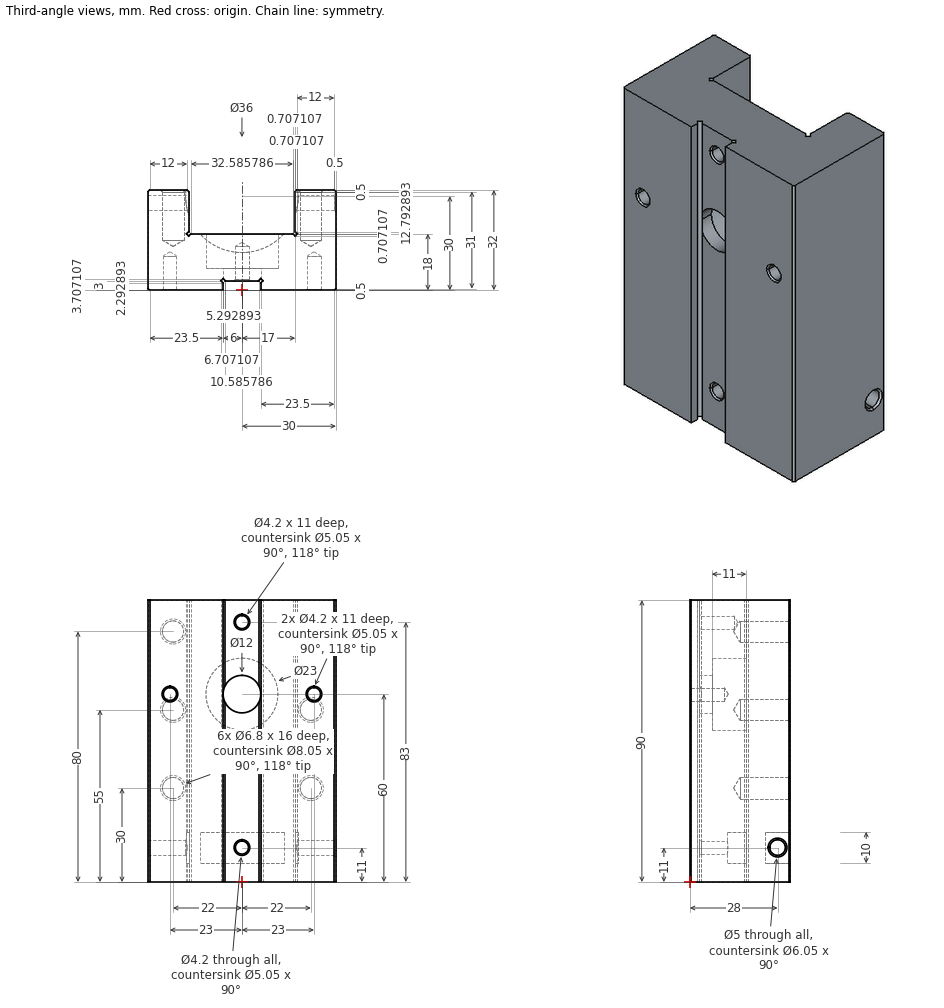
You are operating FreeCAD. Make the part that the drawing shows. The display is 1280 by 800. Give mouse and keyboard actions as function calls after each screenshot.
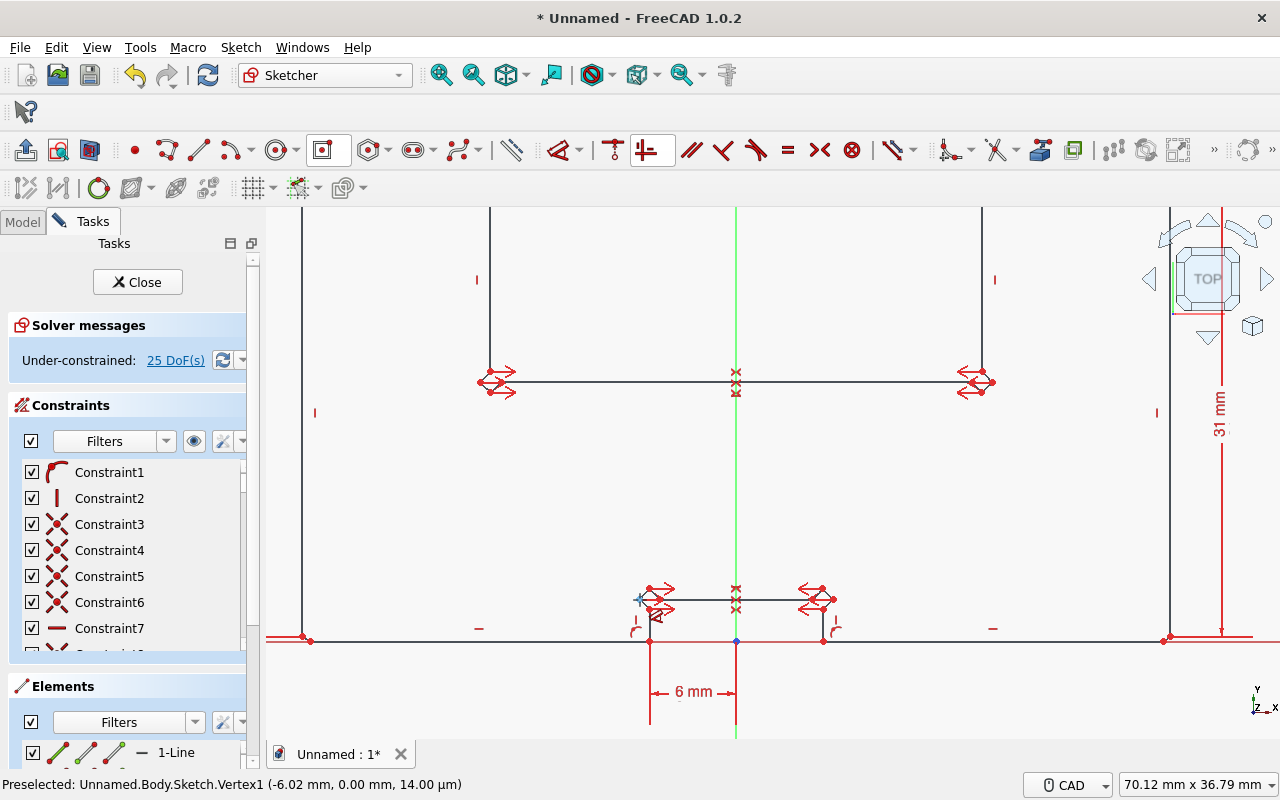
click(640, 600)
click(606, 621)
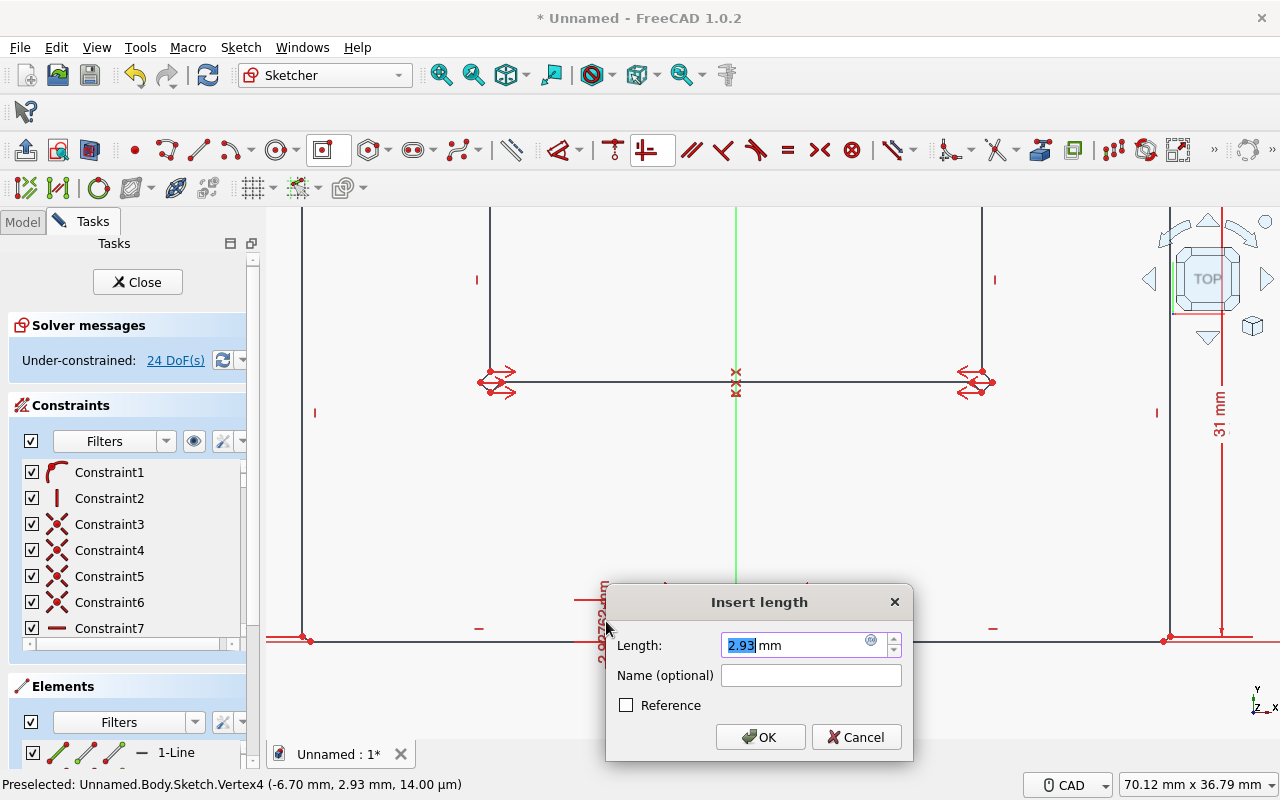
text(3)
key(Return)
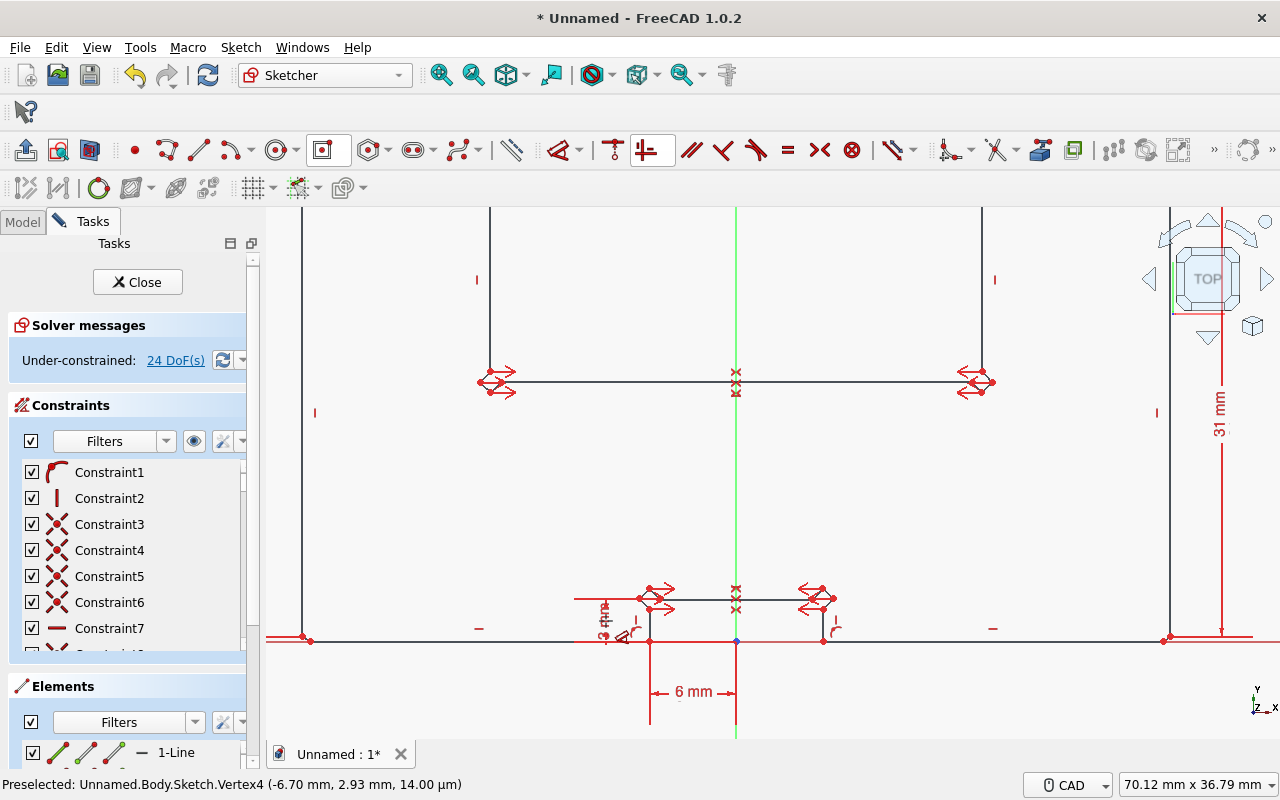
click(650, 589)
click(693, 555)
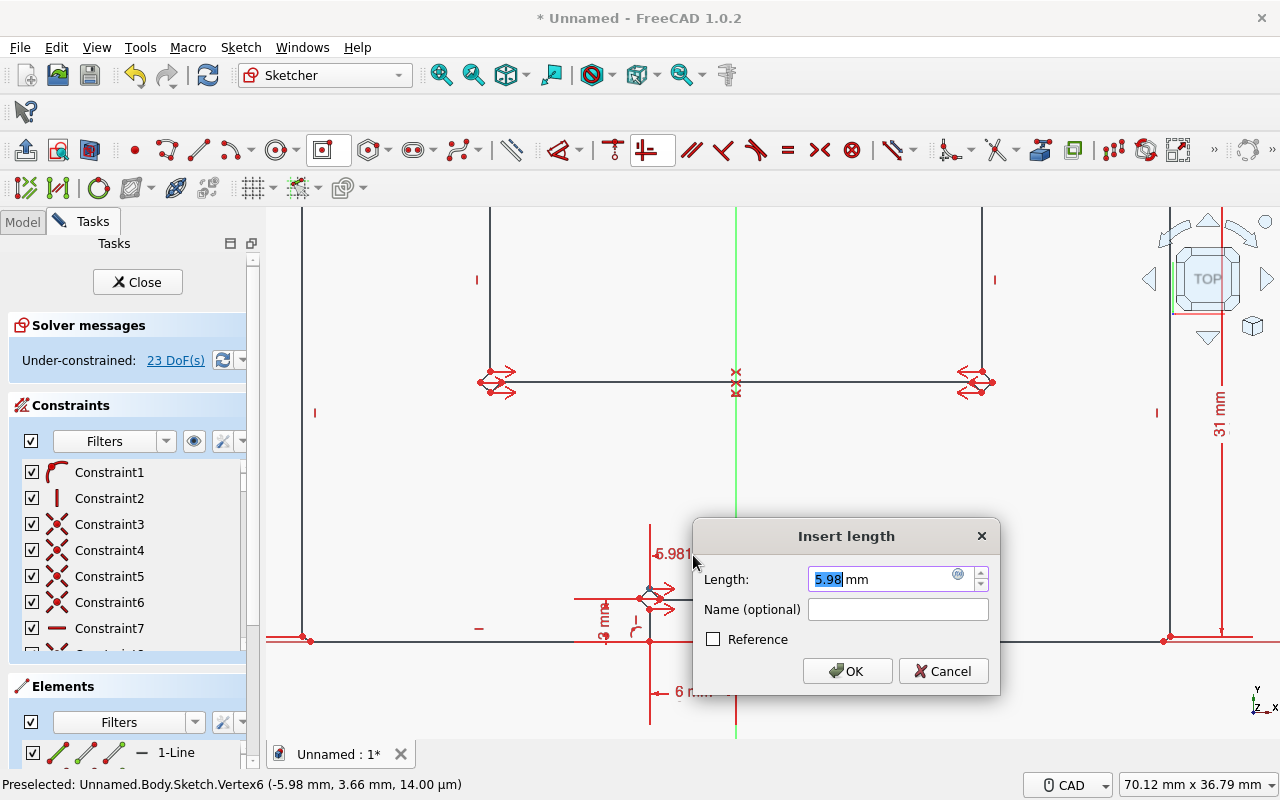
text(6)
key(Return)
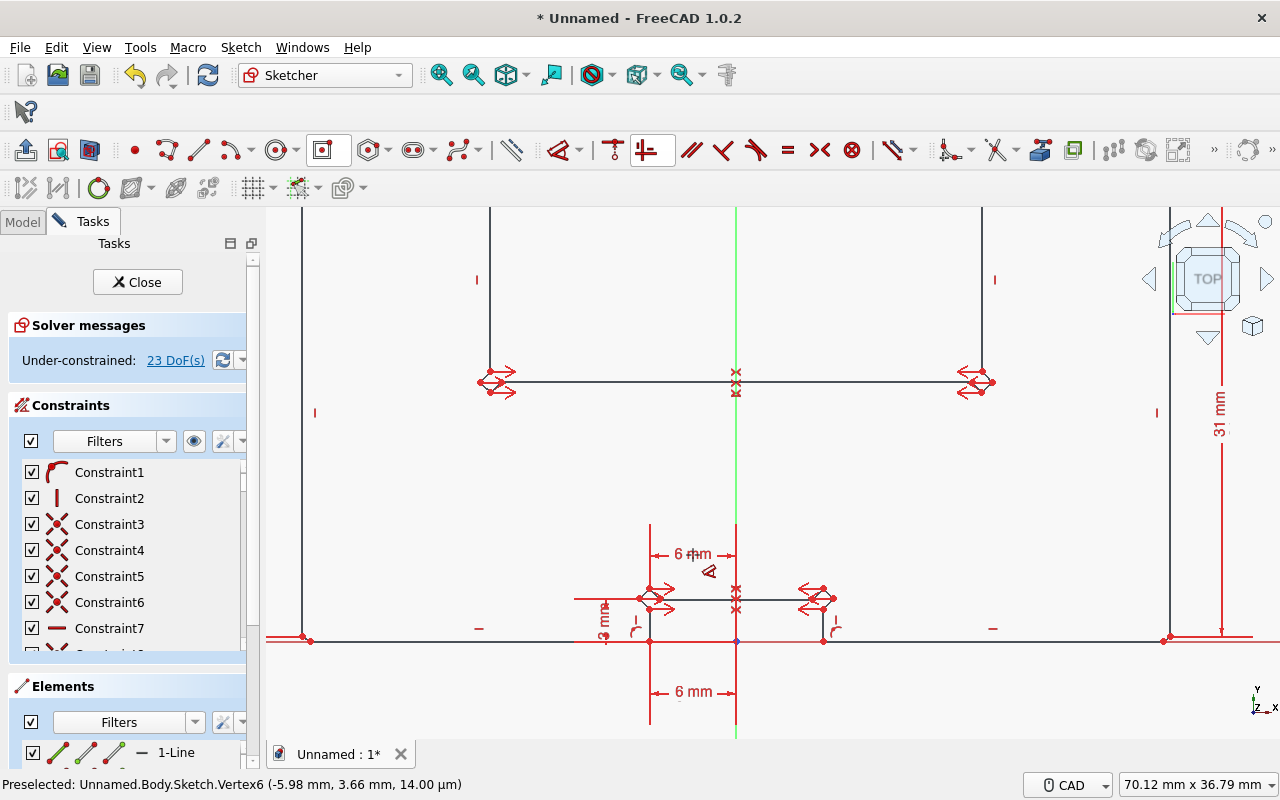
click(660, 600)
click(770, 621)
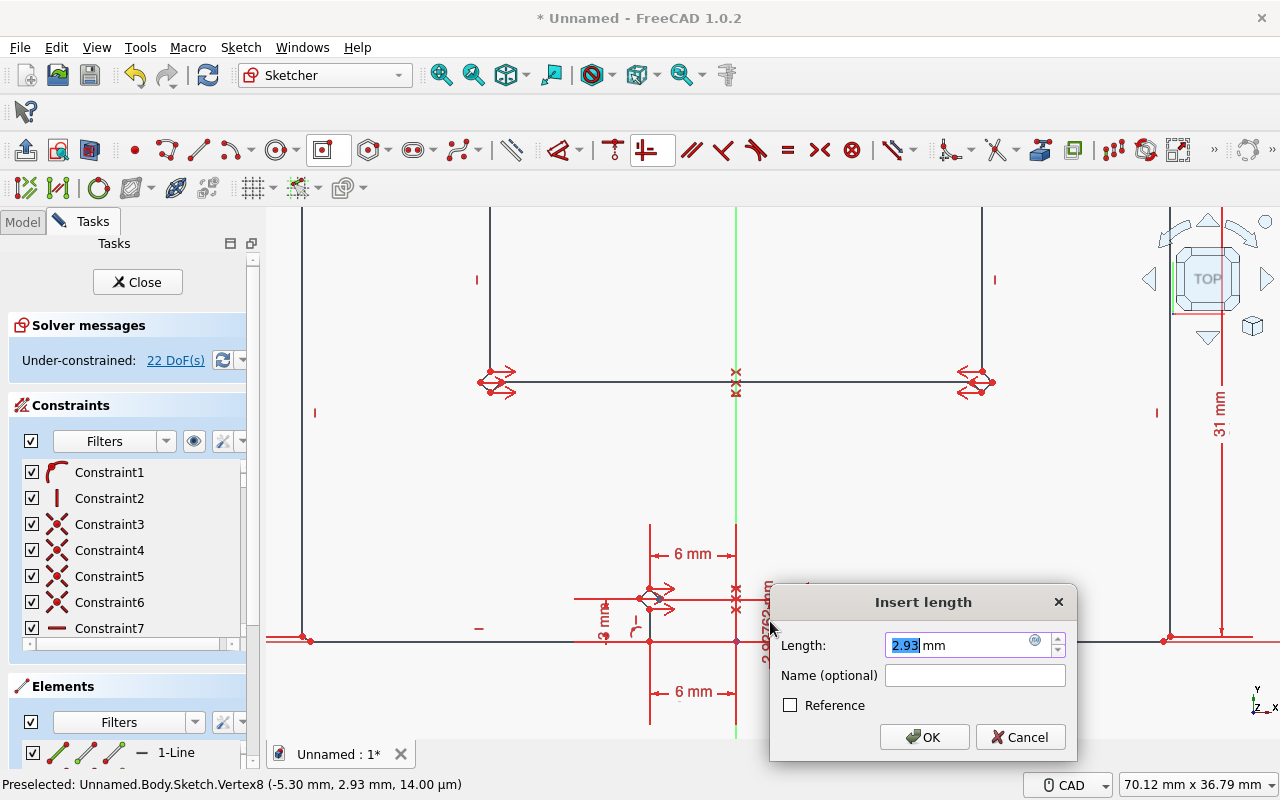
text(3)
key(Return)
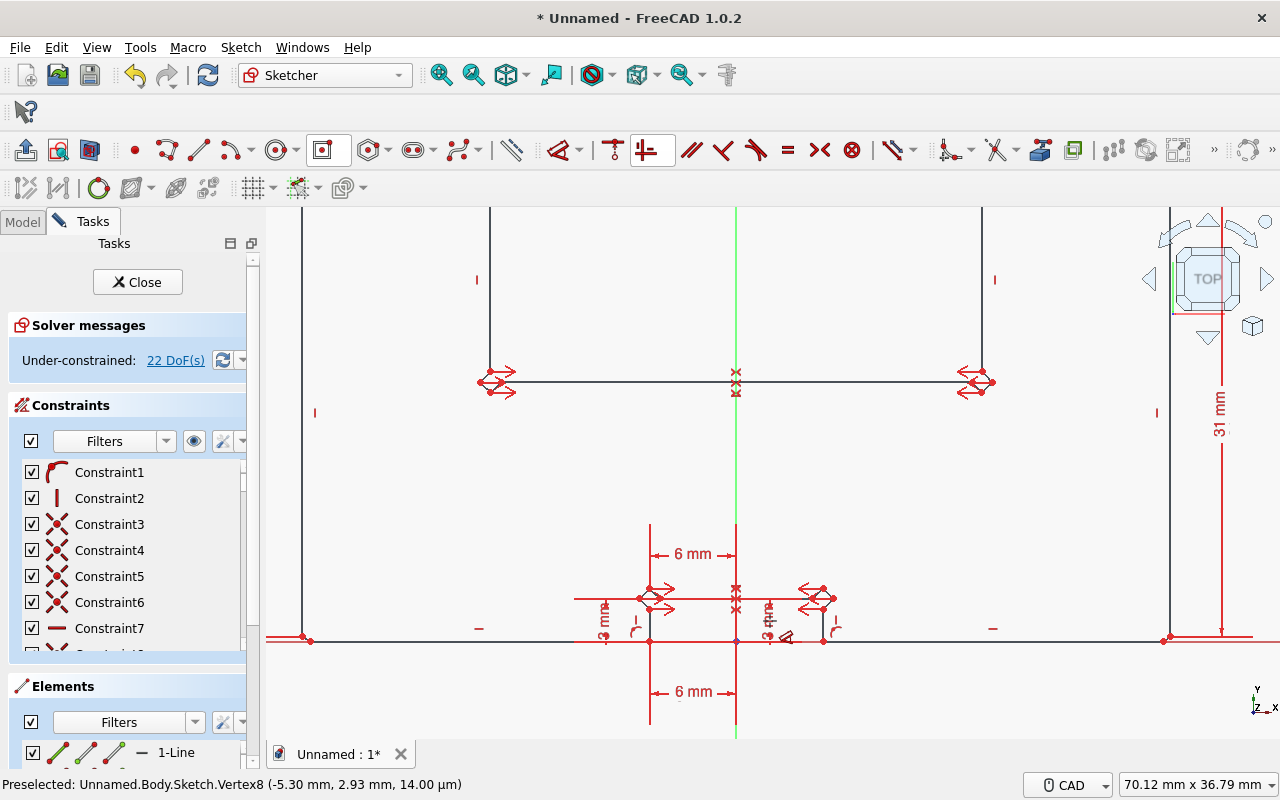
scroll(640, 600, down, 2)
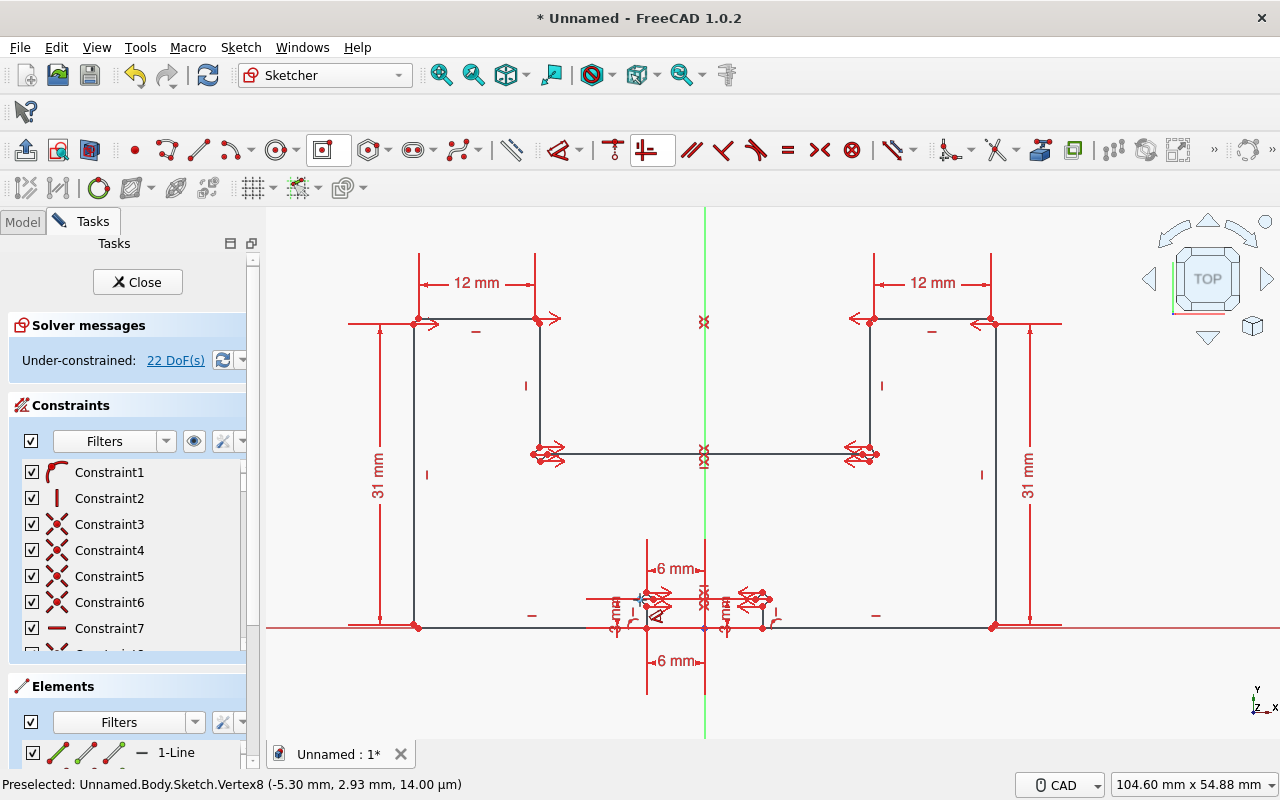
scroll(996, 625, up, 4)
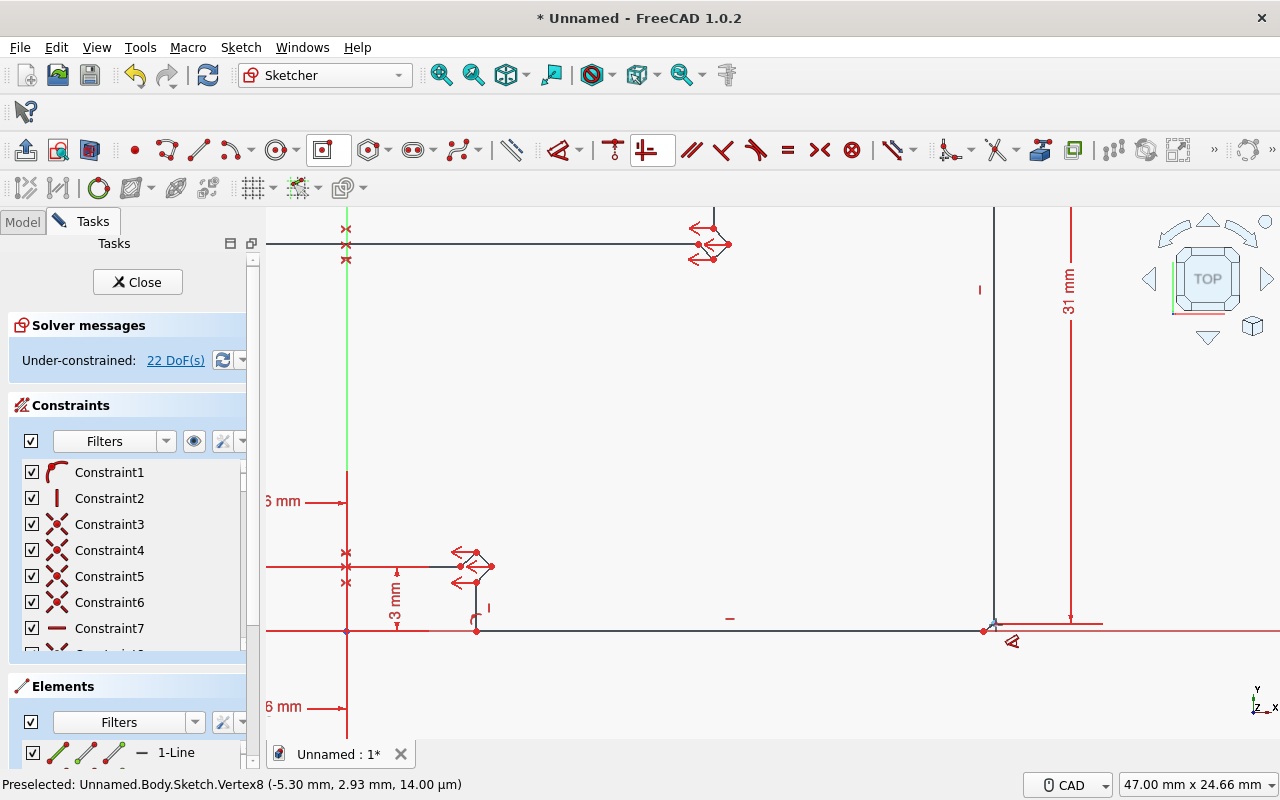
click(994, 624)
click(671, 665)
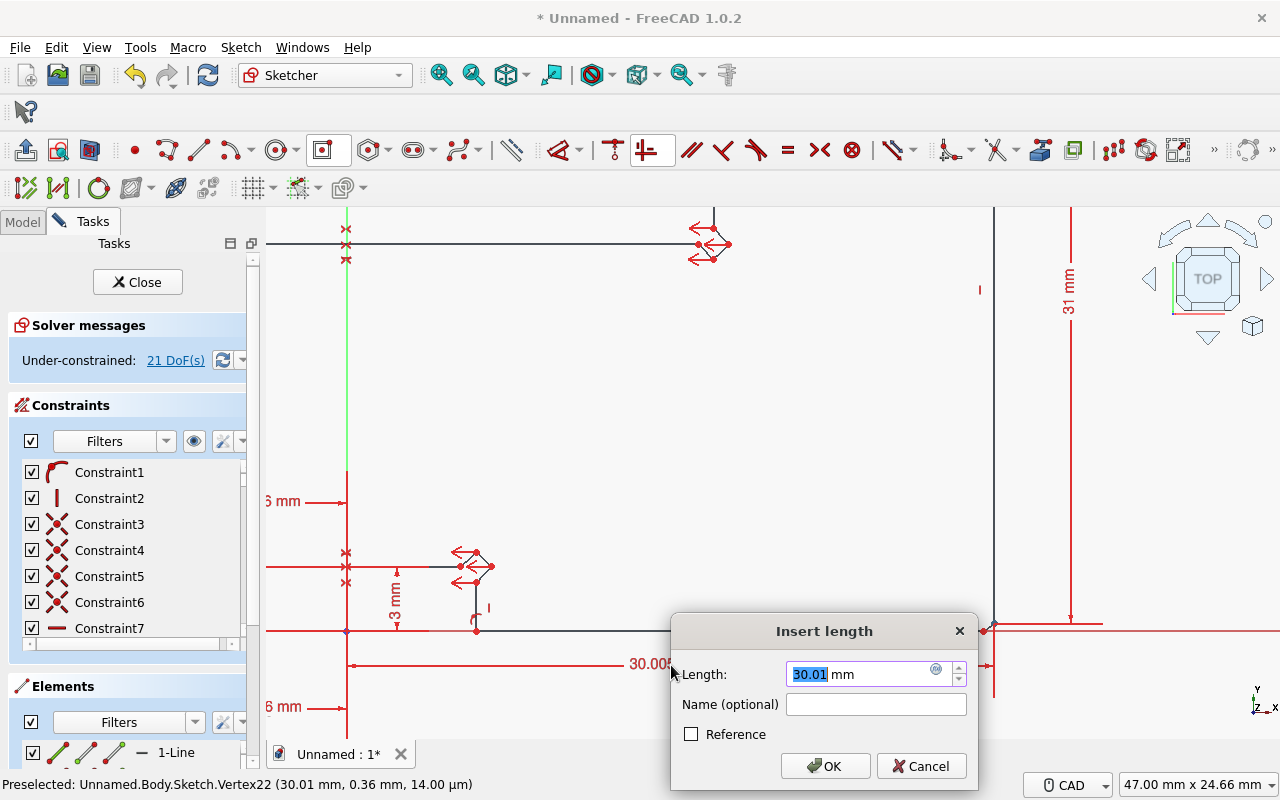
text(30)
key(Return)